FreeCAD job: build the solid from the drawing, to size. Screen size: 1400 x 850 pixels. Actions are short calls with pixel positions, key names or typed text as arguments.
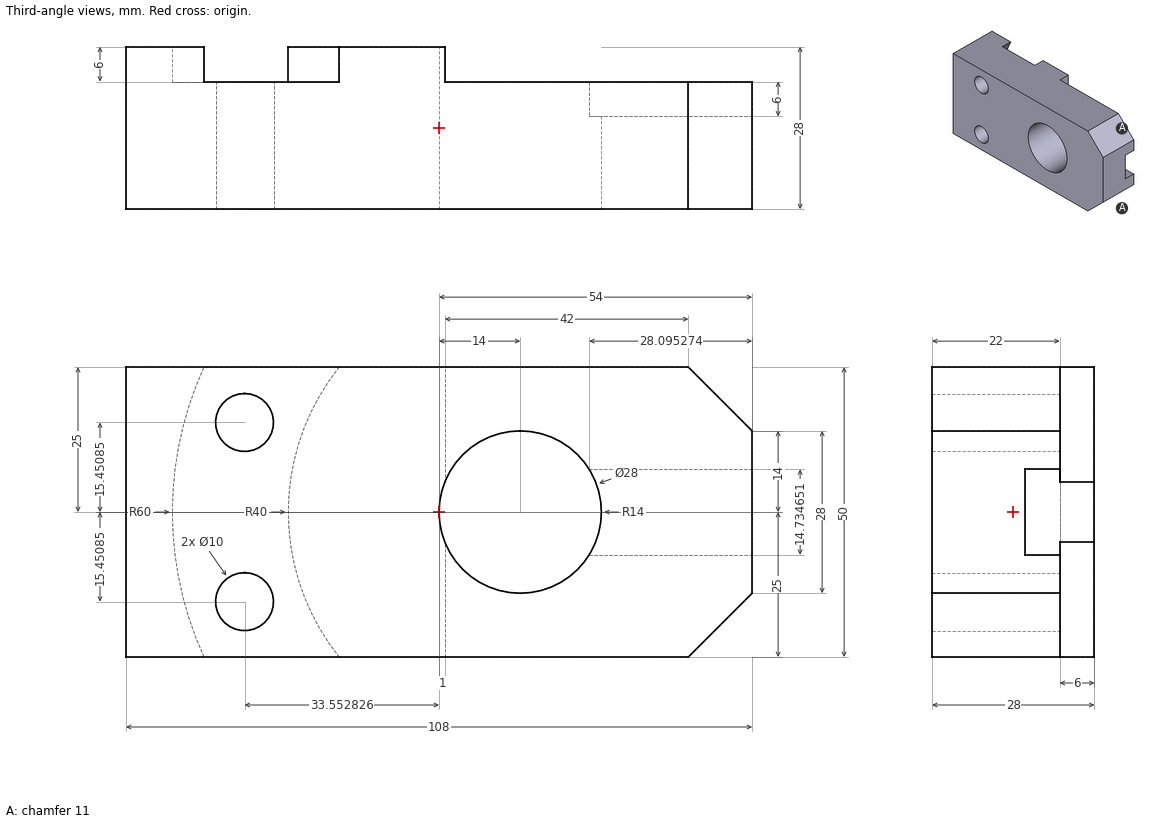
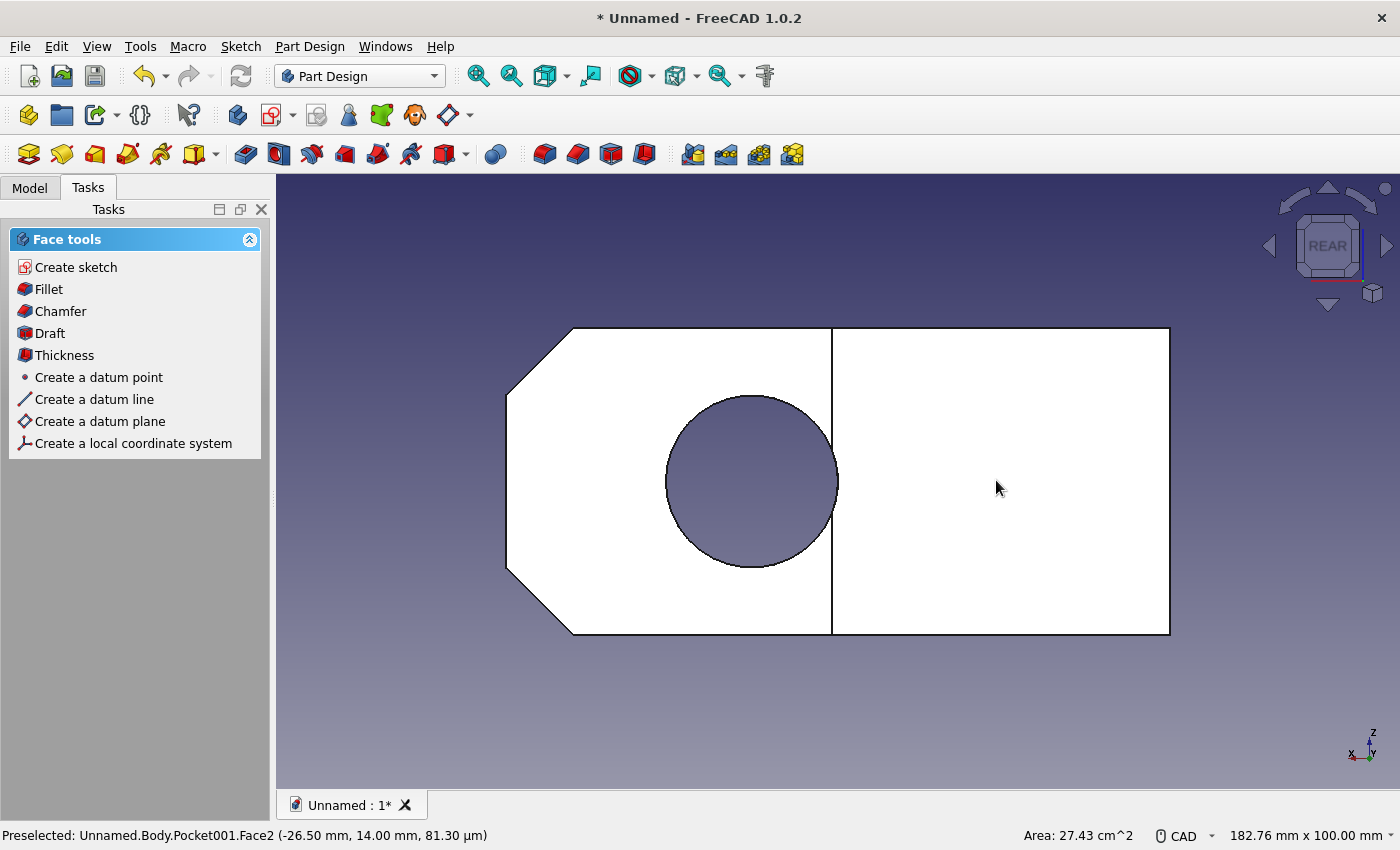
click(270, 116)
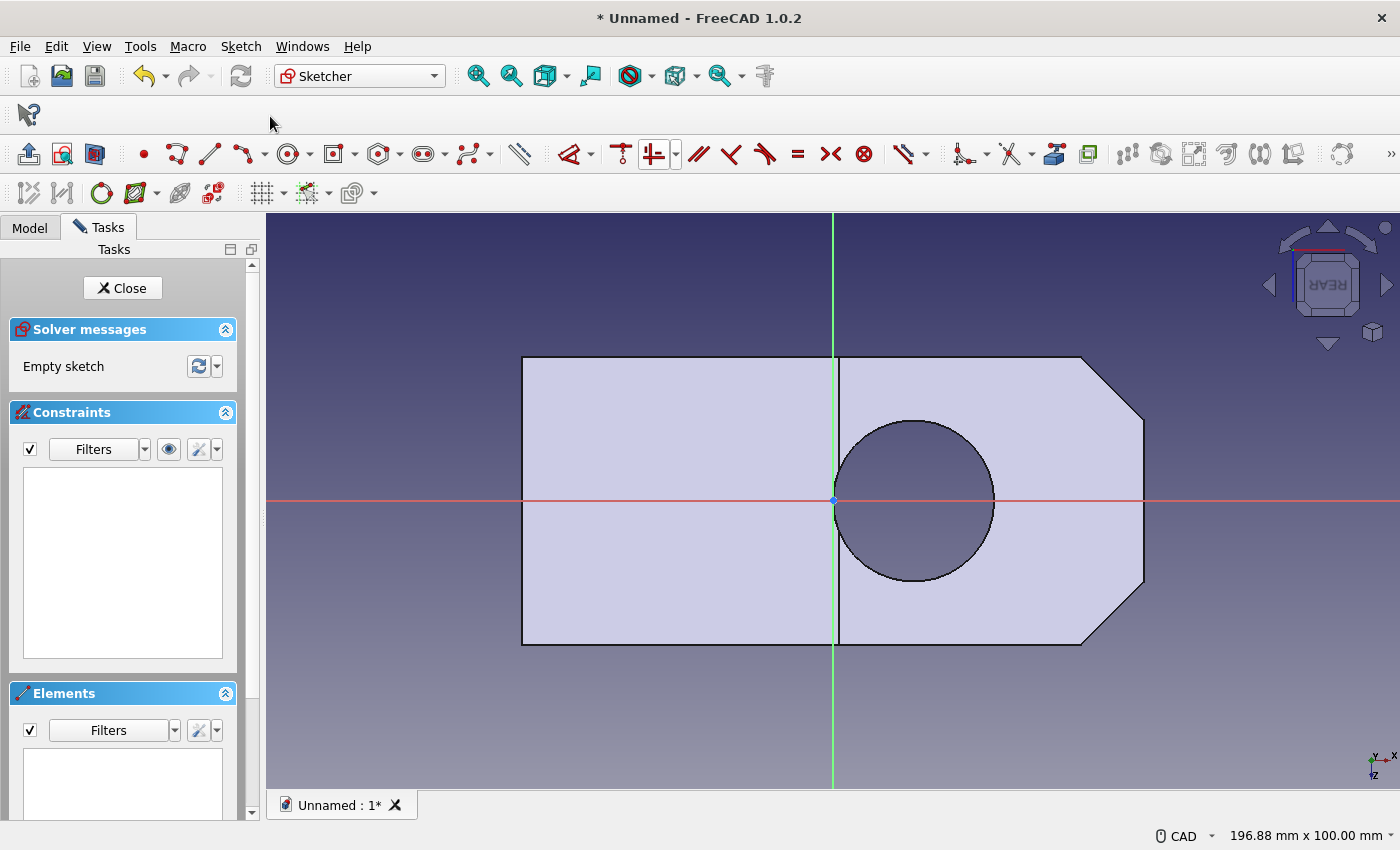
click(210, 154)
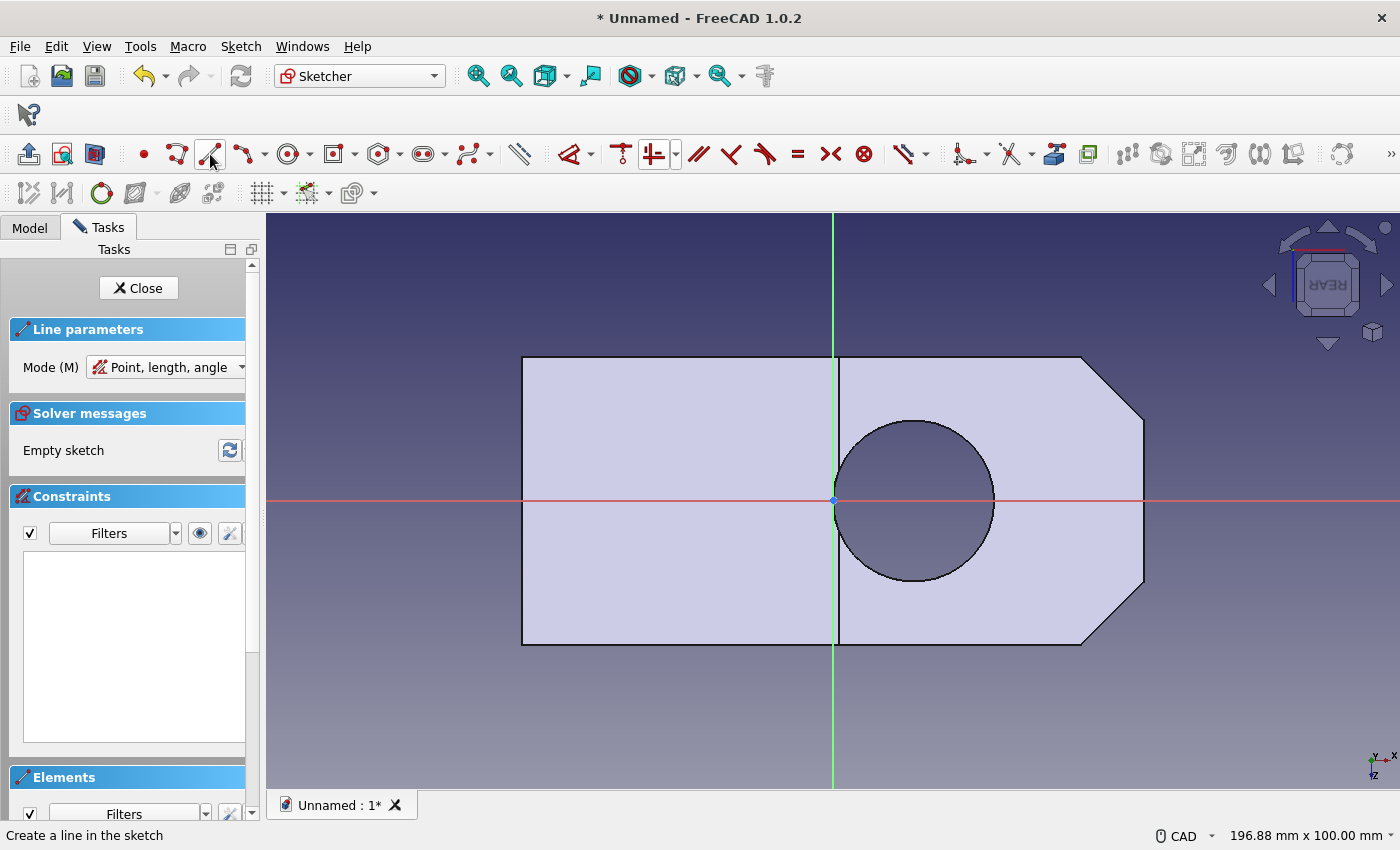
click(599, 645)
click(734, 645)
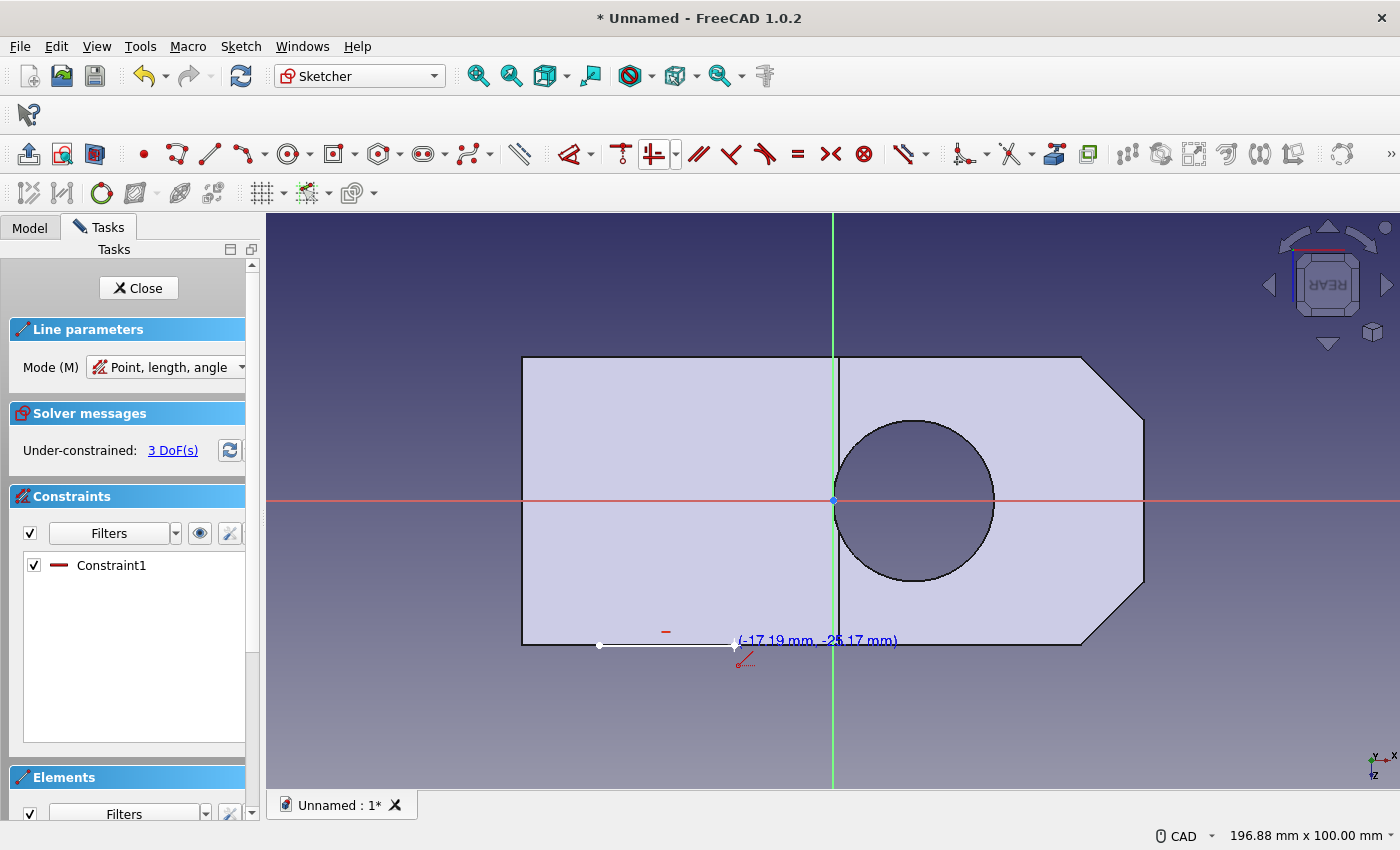
click(734, 357)
click(599, 357)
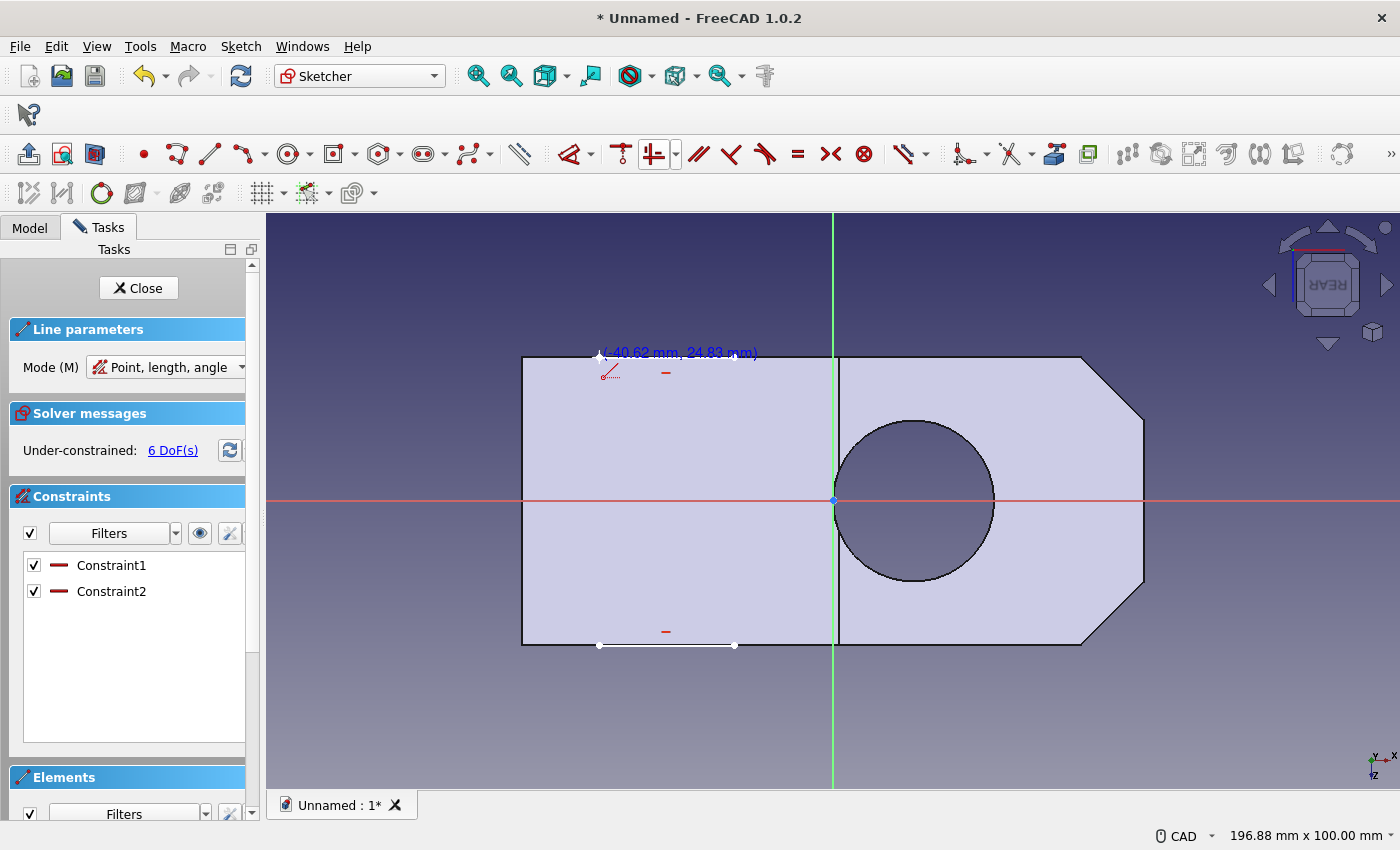
key(g)
key(3)
key(a)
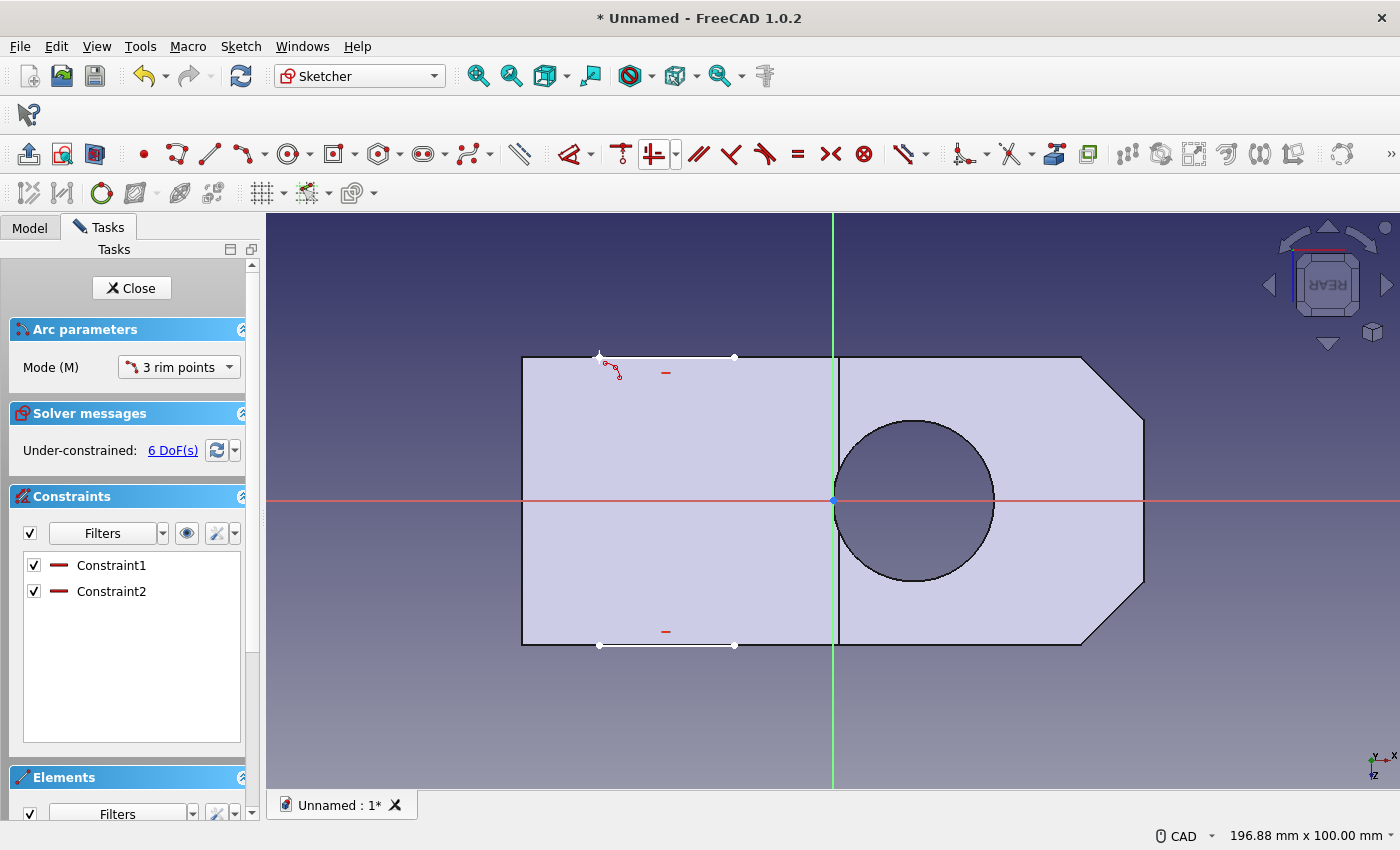
click(734, 646)
click(734, 358)
click(685, 470)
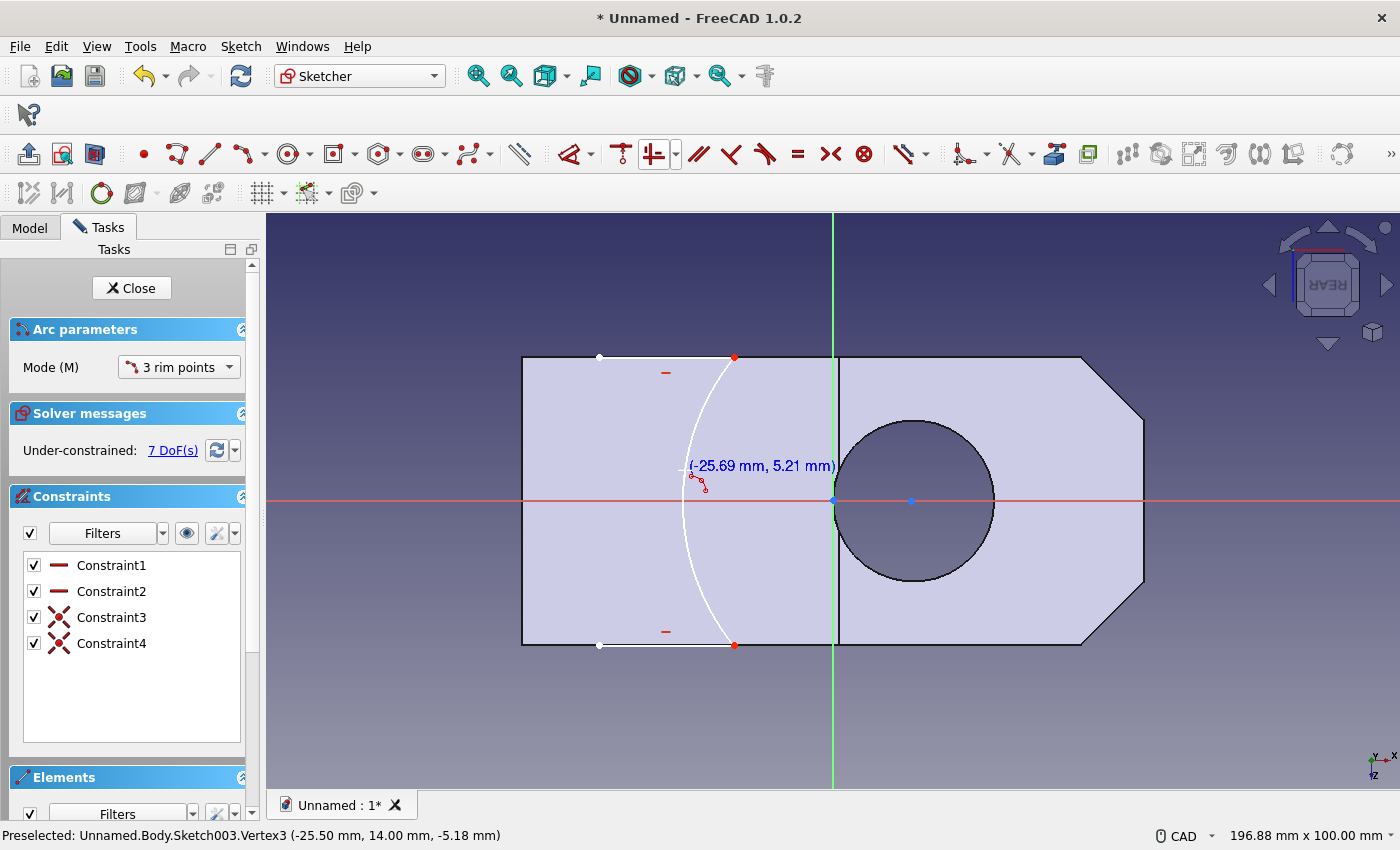
click(599, 358)
click(599, 646)
click(569, 471)
key(Escape)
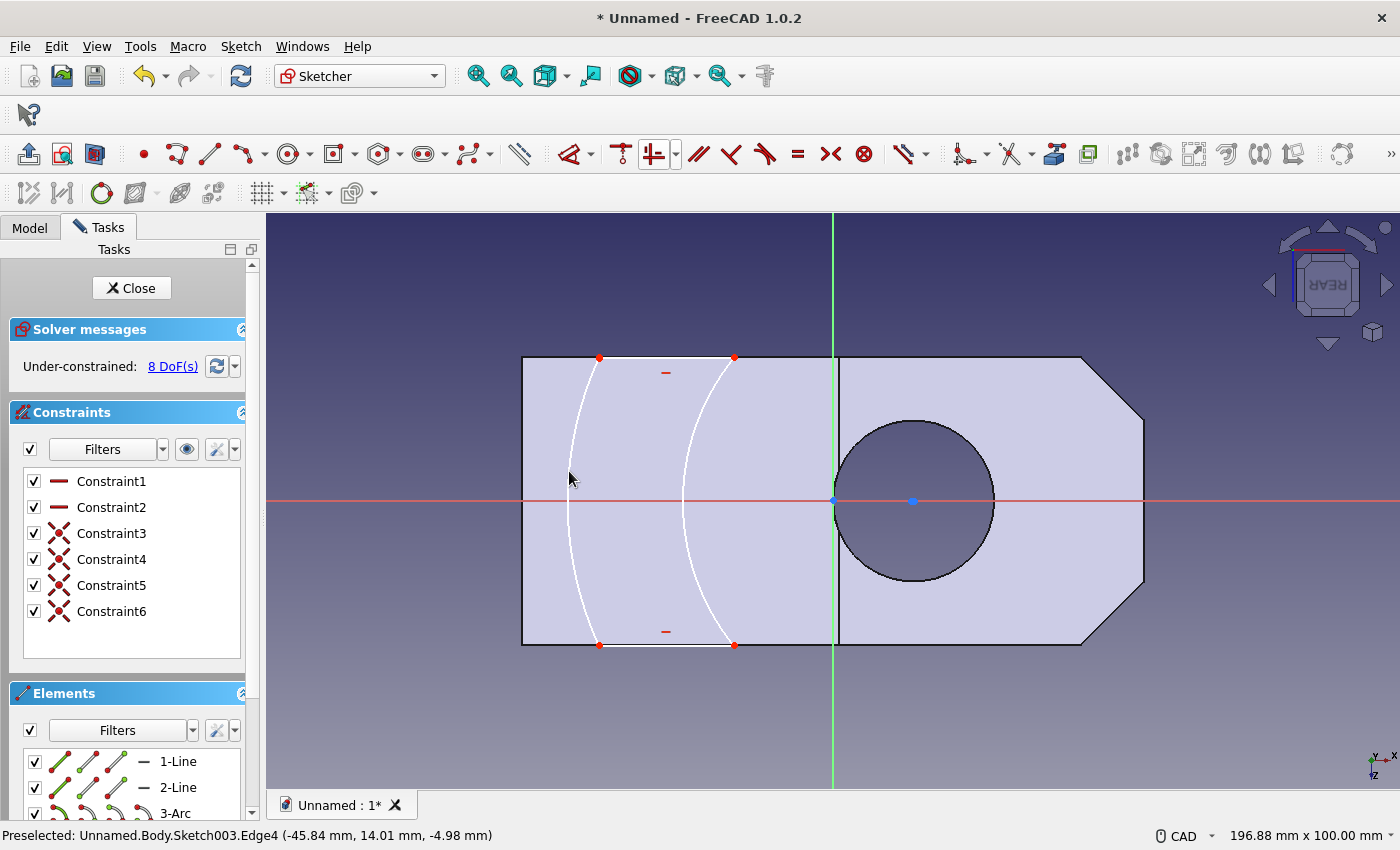
click(691, 440)